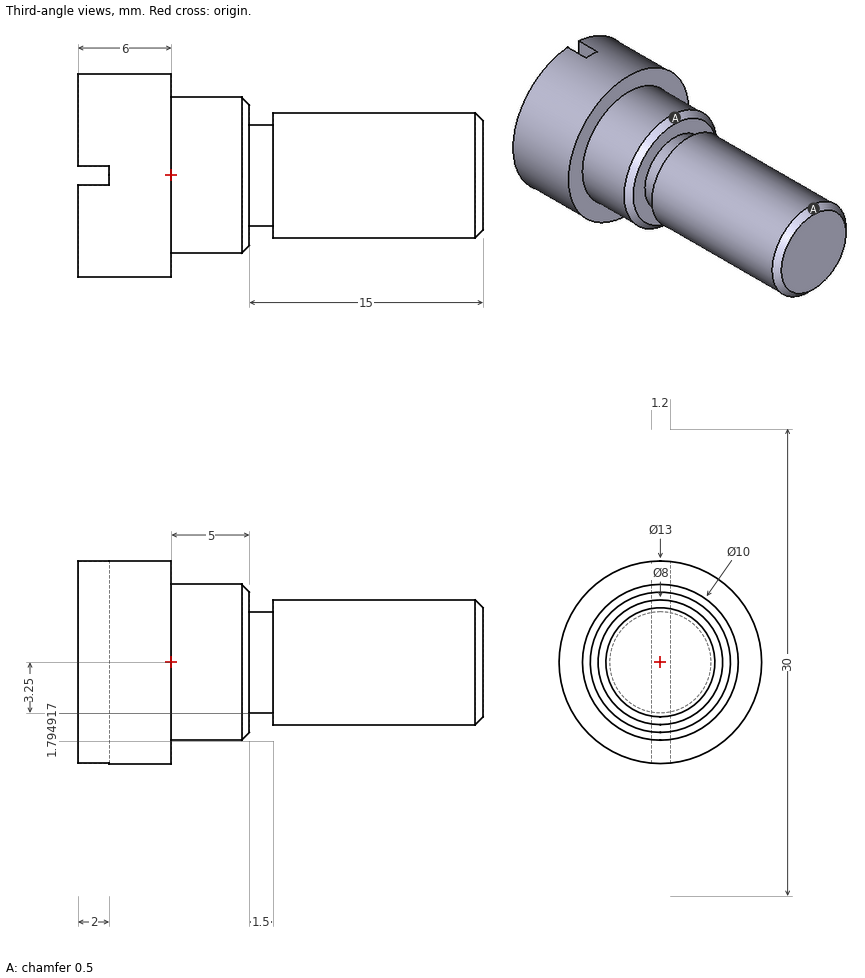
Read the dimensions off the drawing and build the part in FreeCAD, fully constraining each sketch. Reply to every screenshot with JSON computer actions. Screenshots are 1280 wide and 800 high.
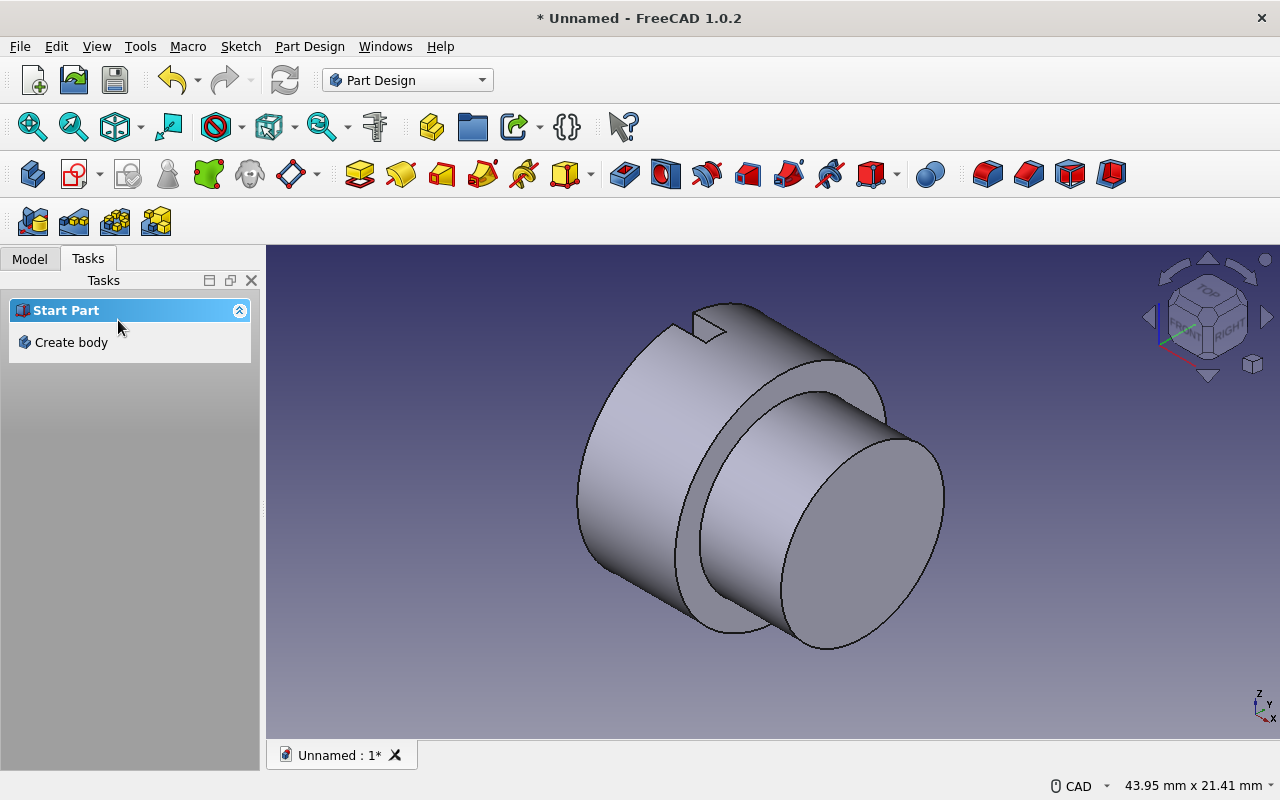
{"action": "left_click", "coordinate": [863, 543]}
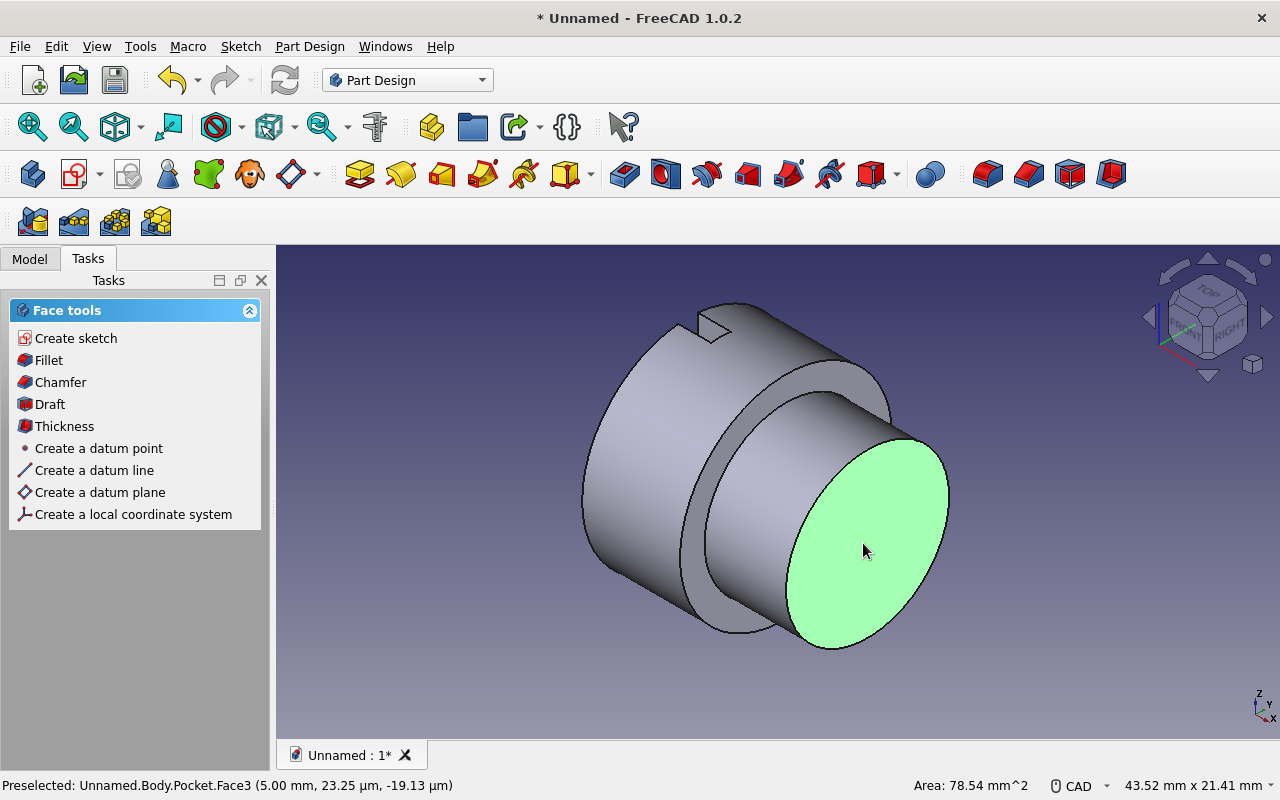
{"action": "left_click", "coordinate": [74, 174]}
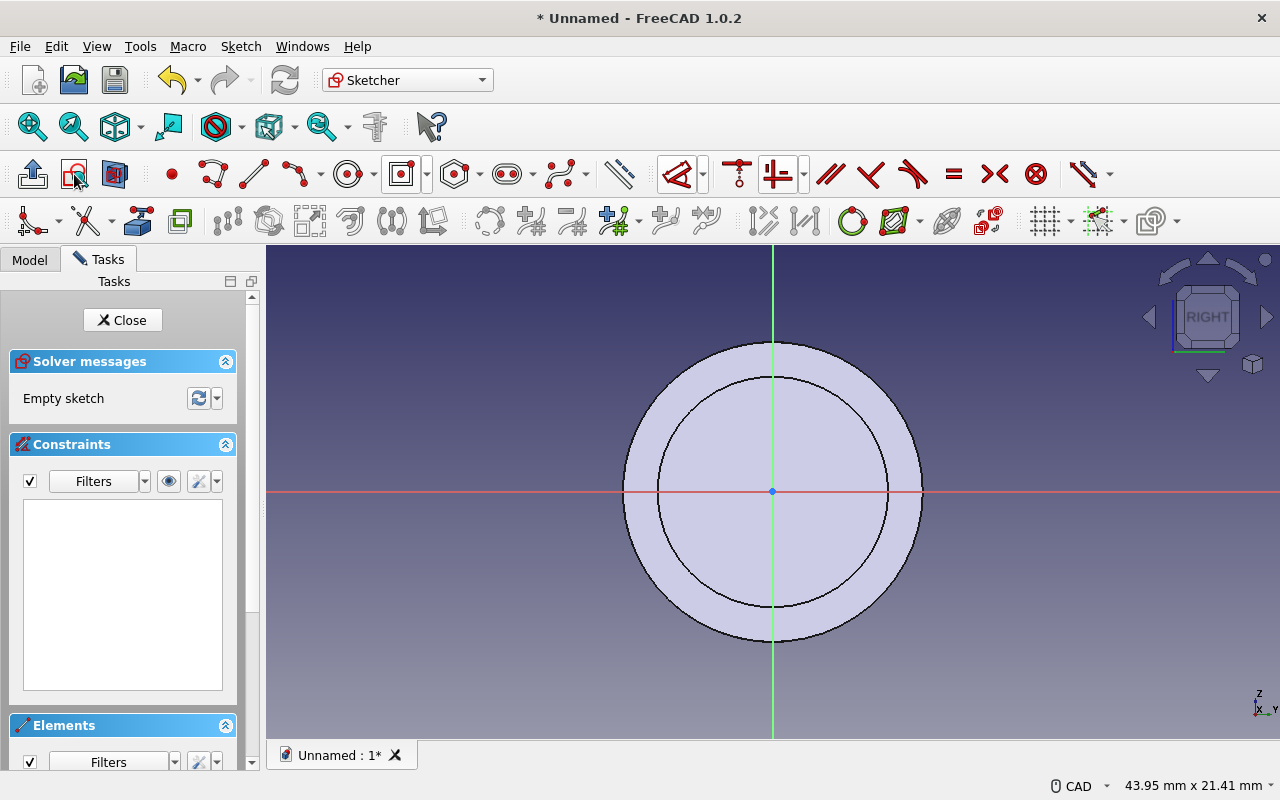
{"action": "scroll", "coordinate": [856, 492], "scroll_direction": "up", "scroll_amount": 3}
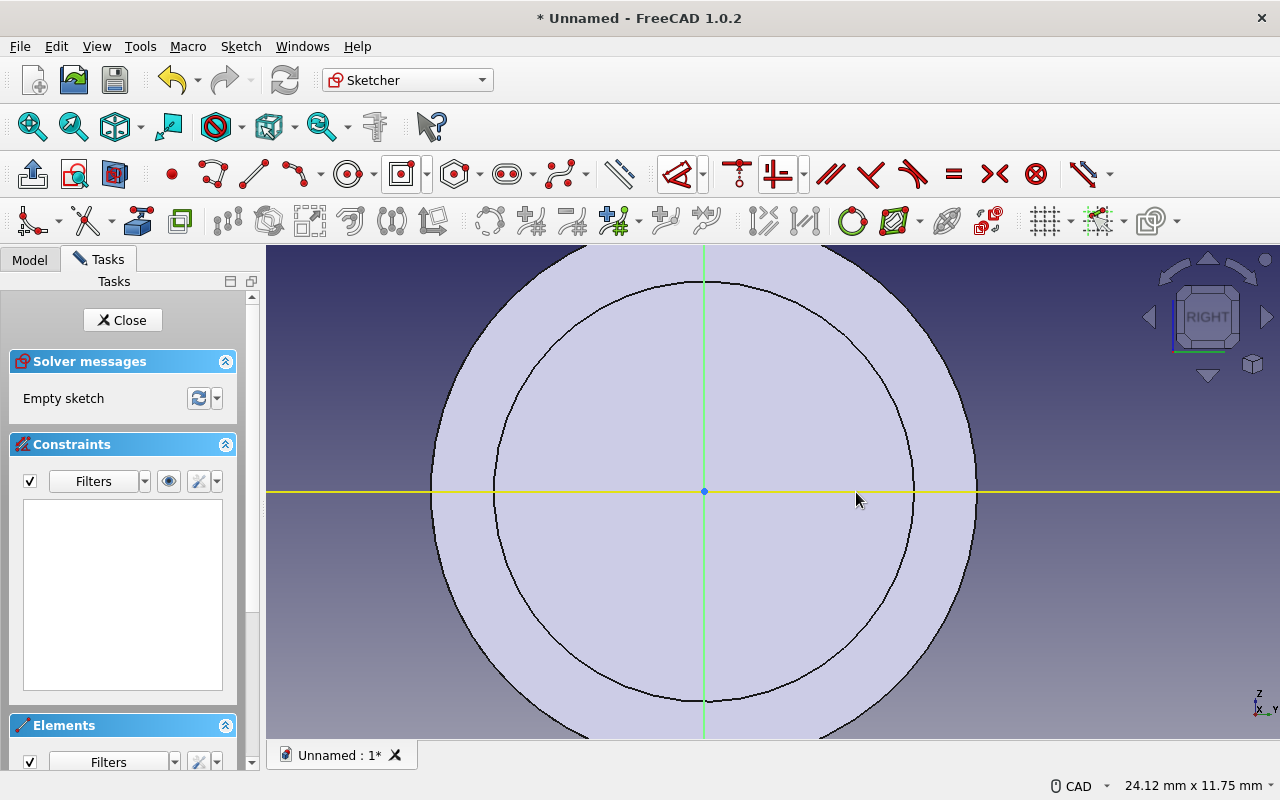
{"action": "left_click", "coordinate": [348, 174]}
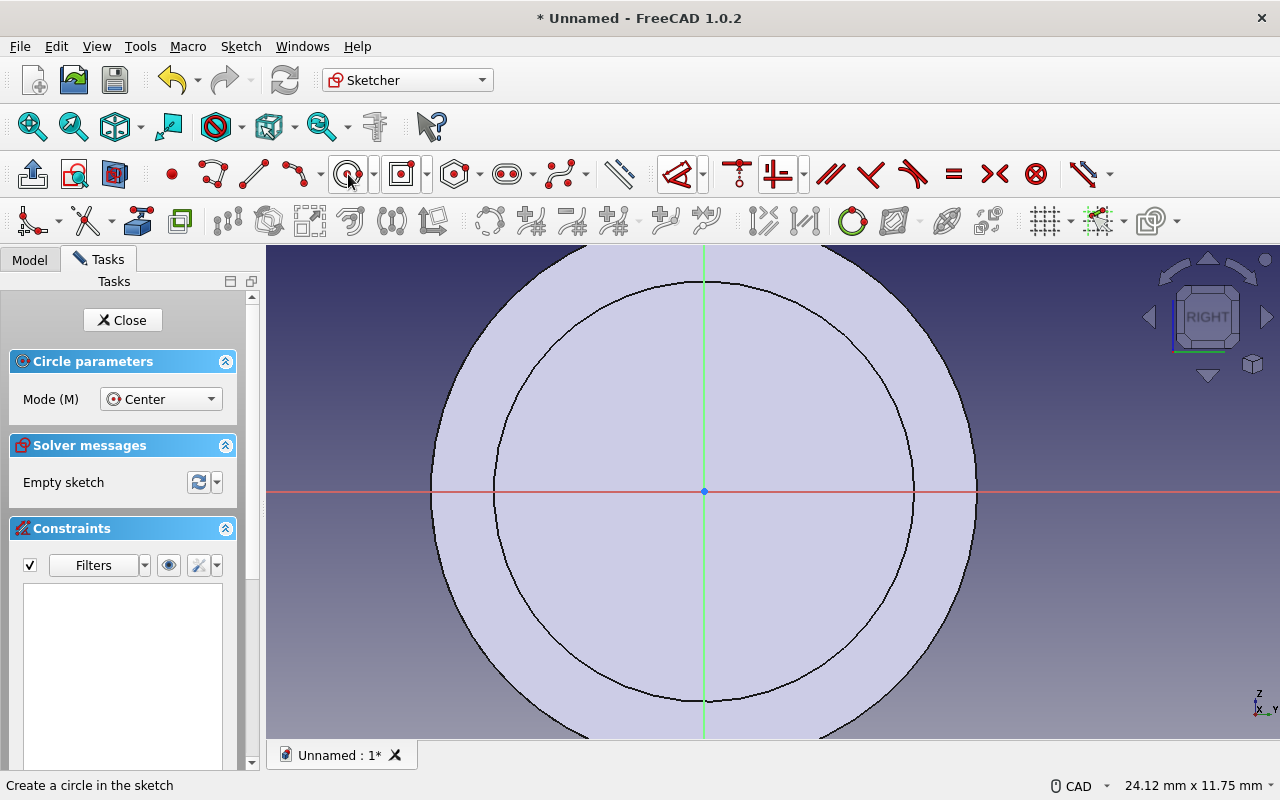
{"action": "left_click", "coordinate": [704, 492]}
{"action": "mouse_move", "coordinate": [823, 373]}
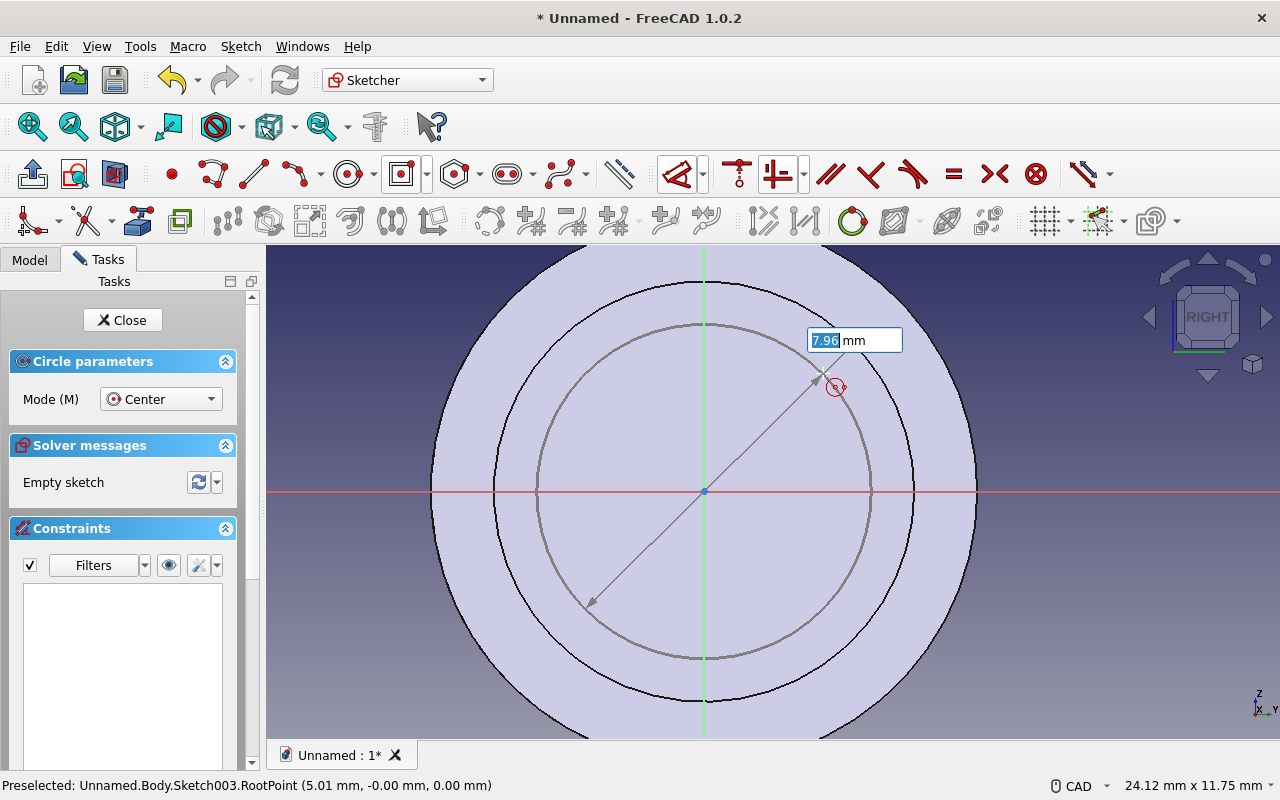
{"action": "type", "text": "8"}
{"action": "key", "text": "Return"}
{"action": "key", "text": "Escape"}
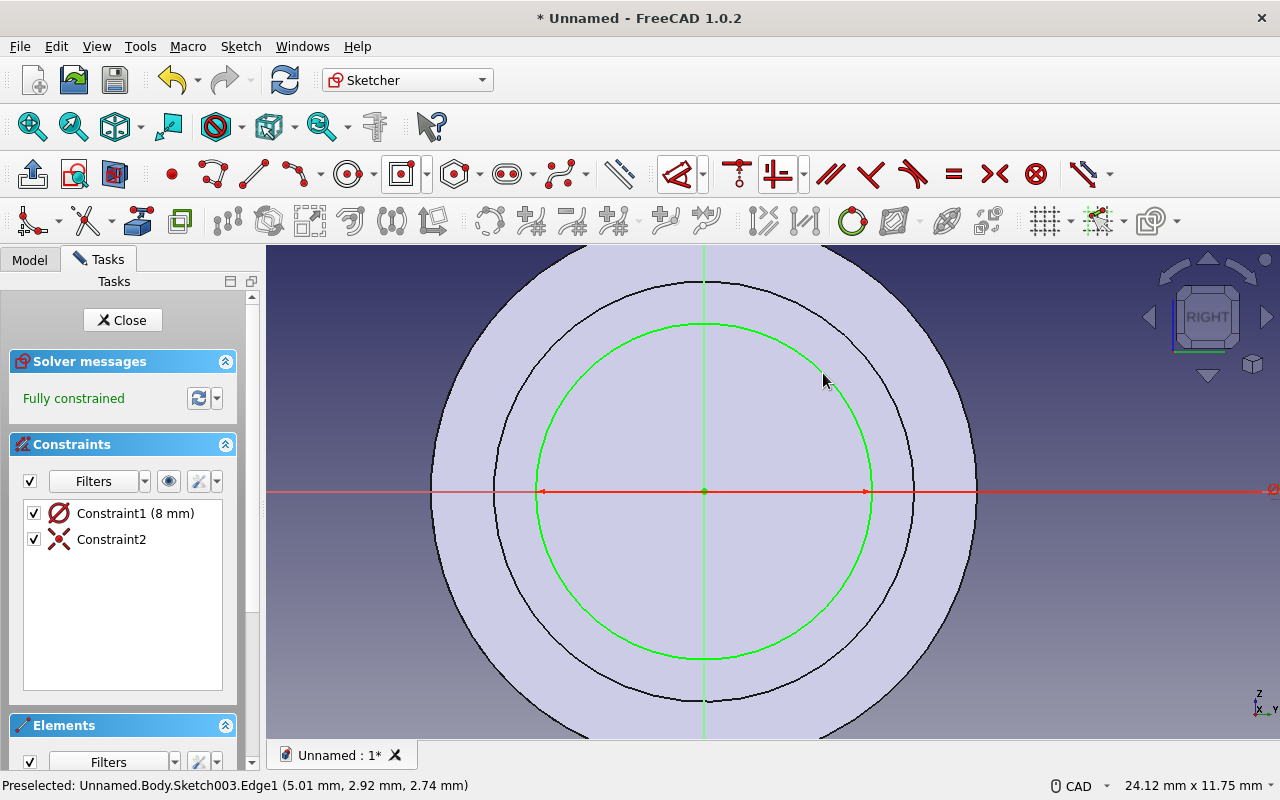
{"action": "left_click", "coordinate": [123, 320]}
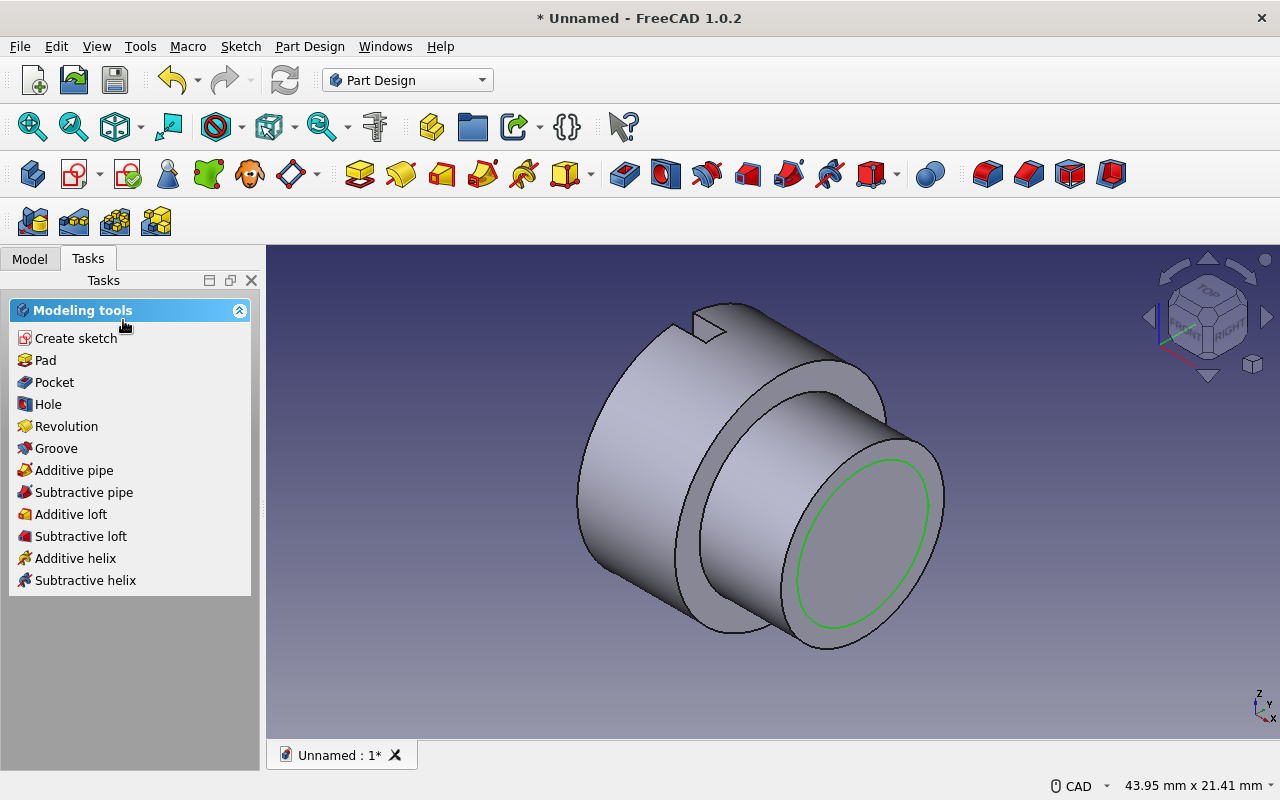
{"action": "left_click", "coordinate": [360, 174]}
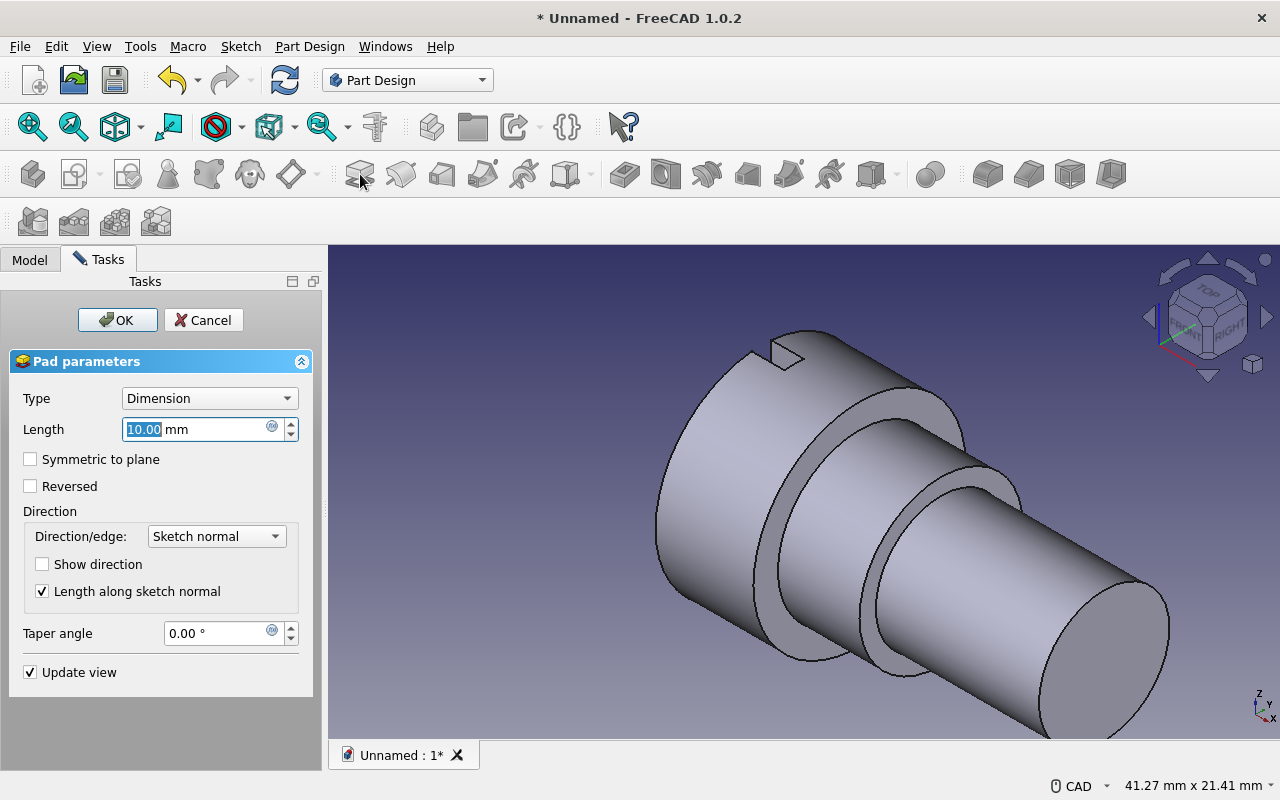
{"action": "type", "text": "15"}
{"action": "key", "text": "Tab"}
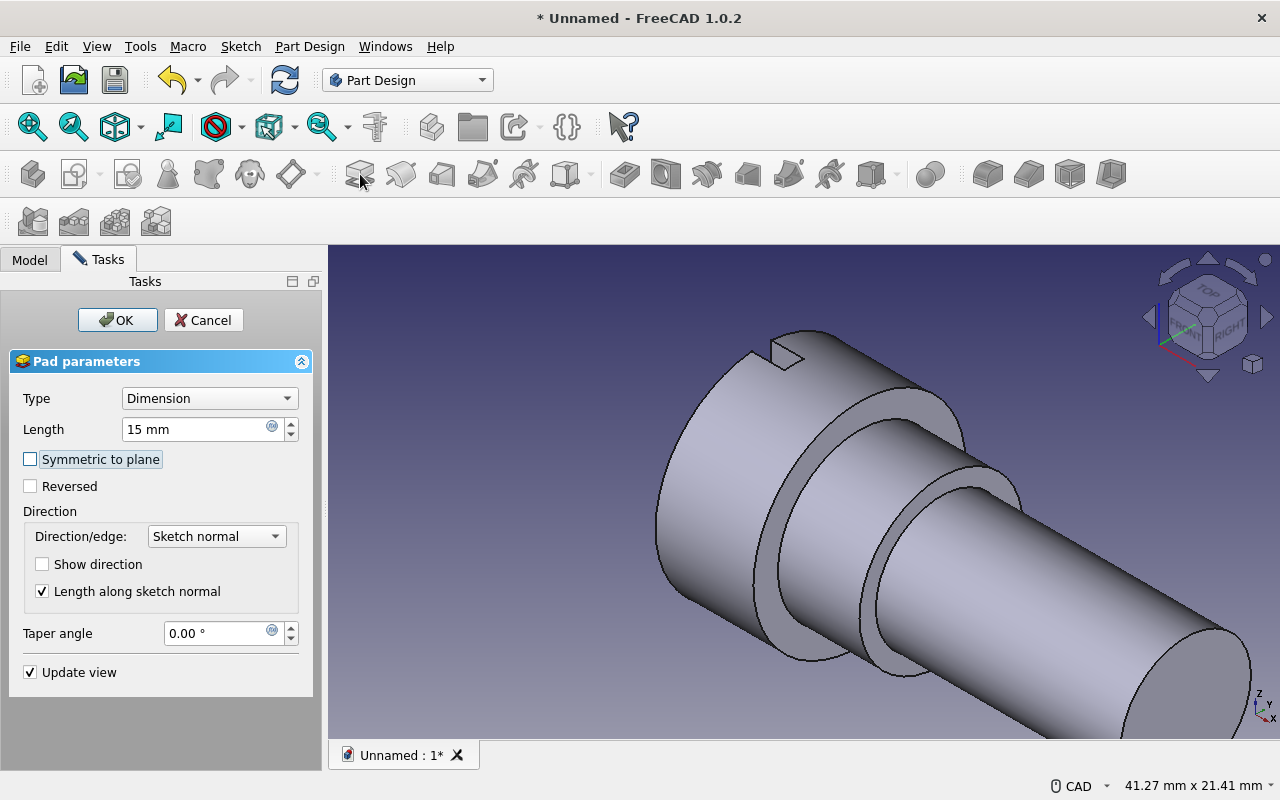
{"action": "left_click", "coordinate": [118, 320]}